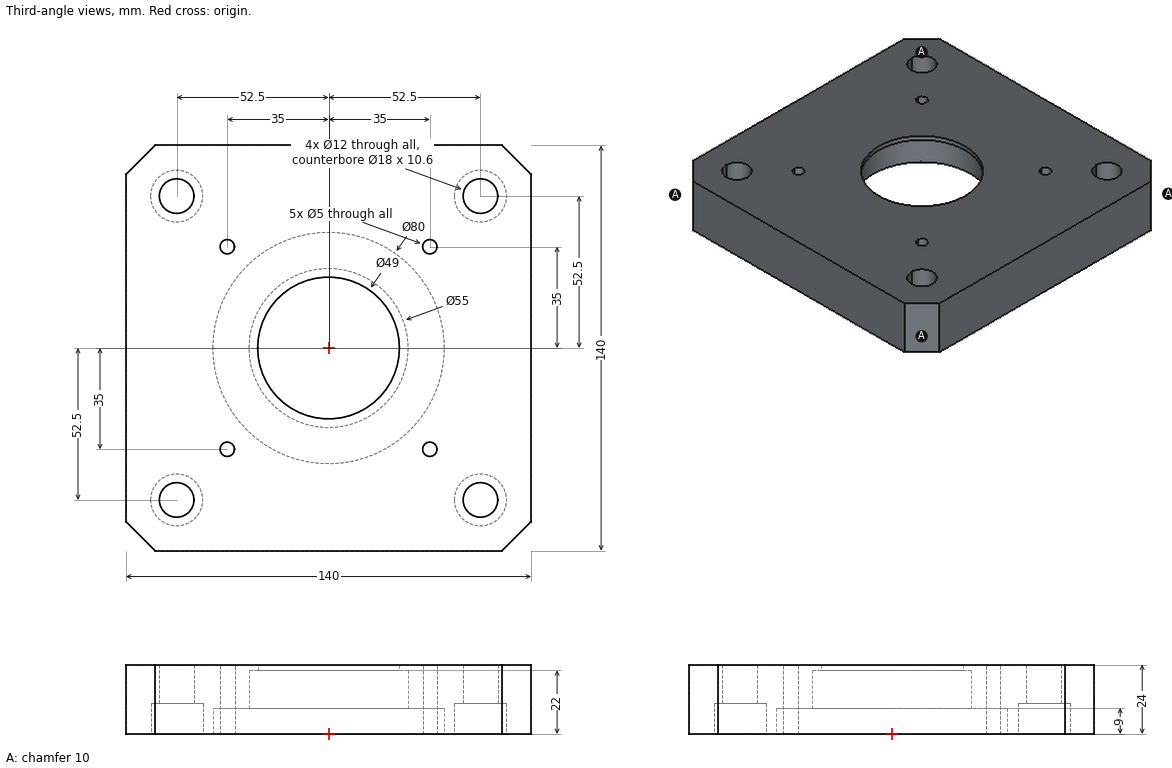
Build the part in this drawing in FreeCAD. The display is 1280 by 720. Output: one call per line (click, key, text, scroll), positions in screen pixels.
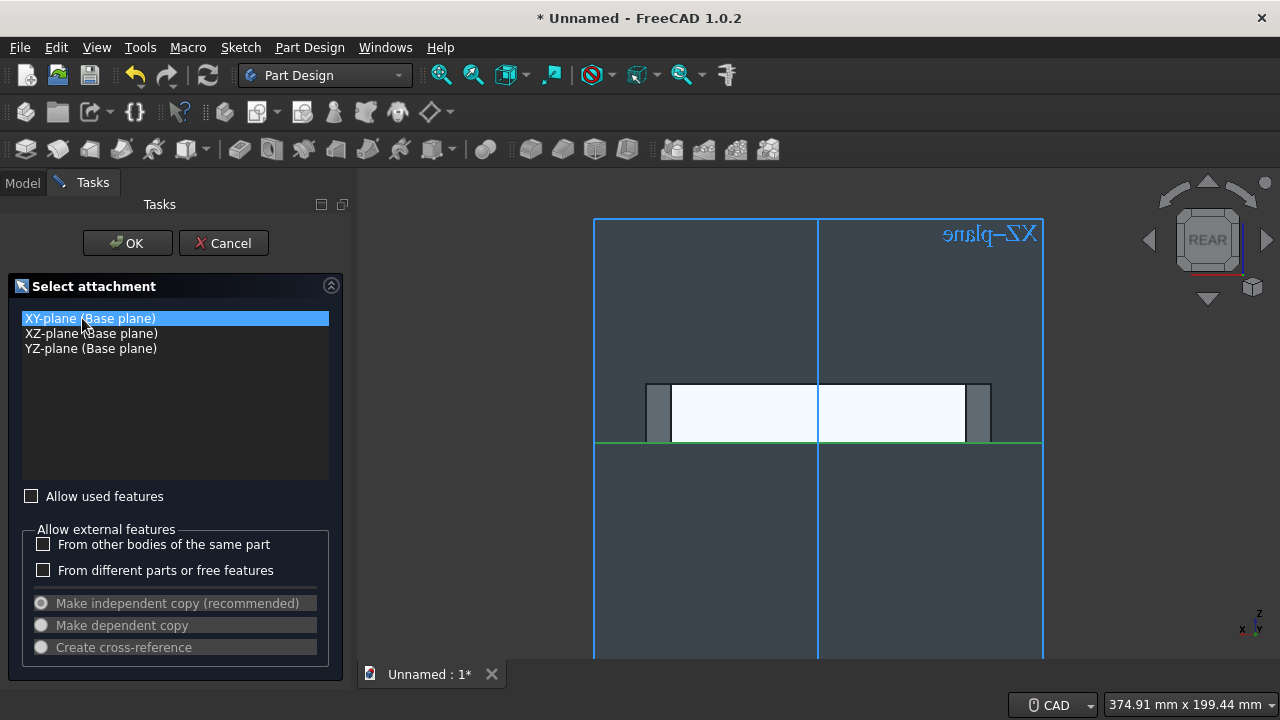
click(128, 243)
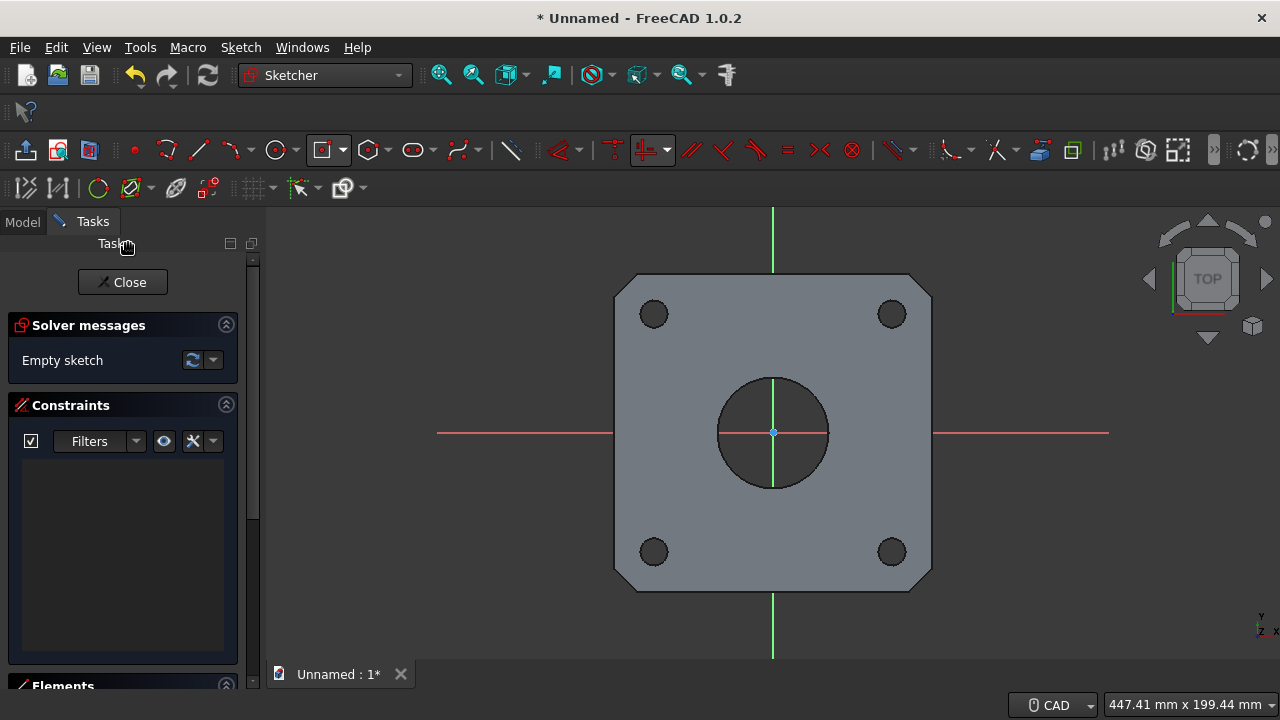
click(90, 150)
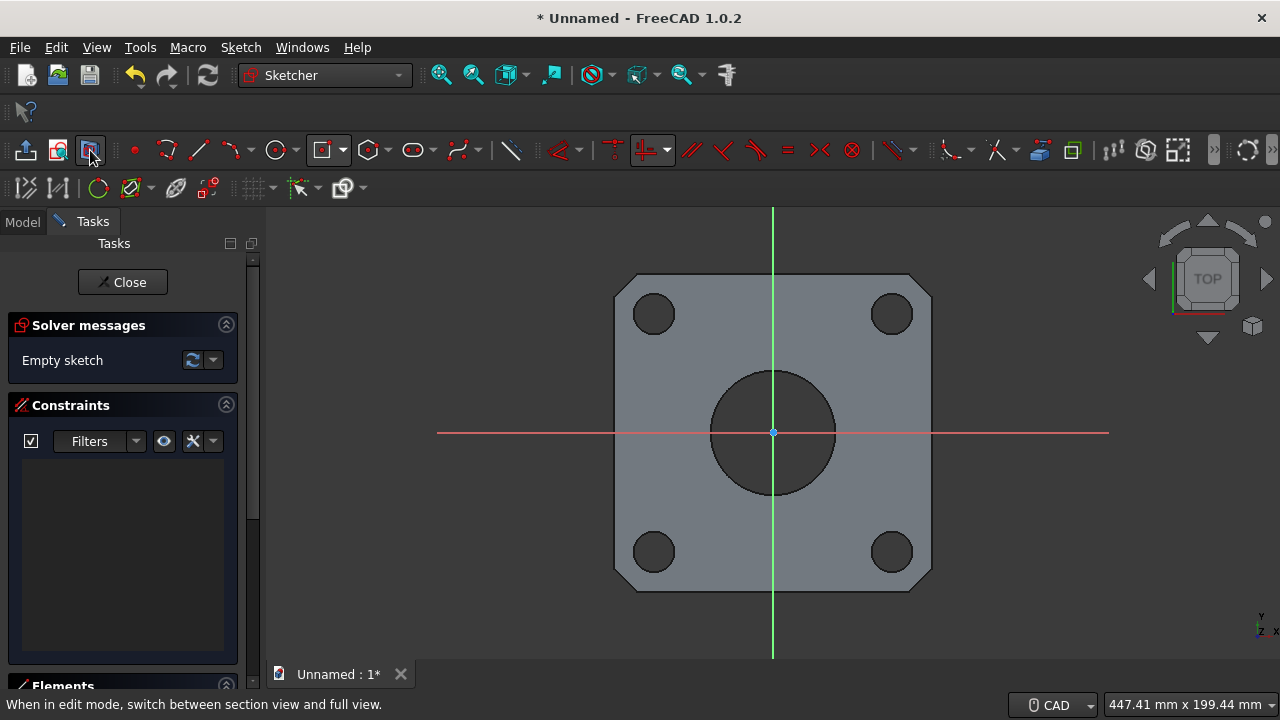
scroll(912, 433, up, 2)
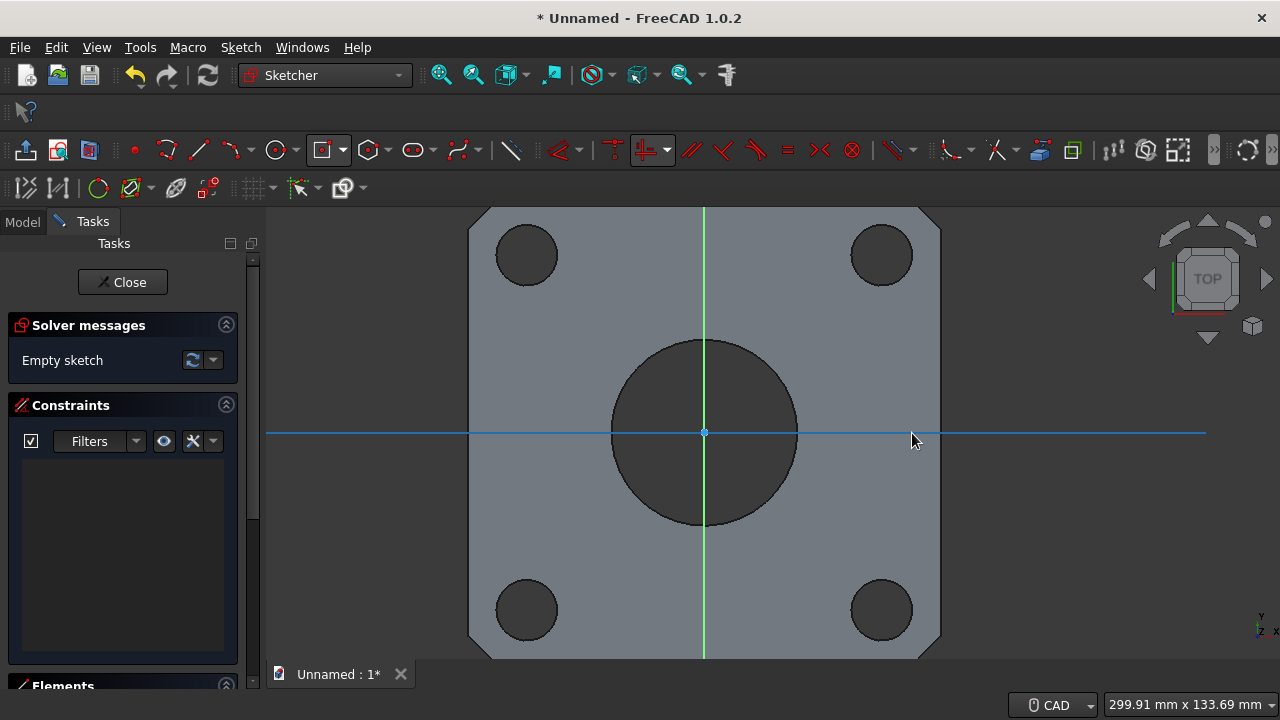
click(276, 150)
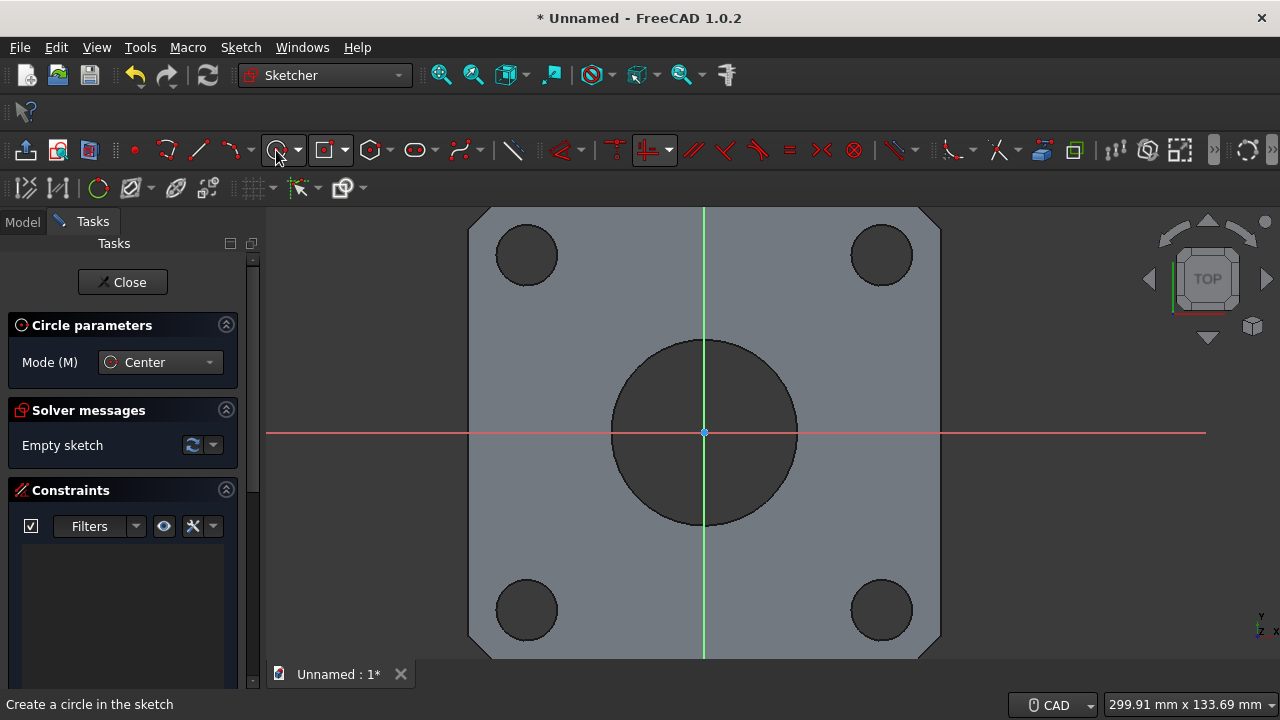
scroll(823, 314, up, 5)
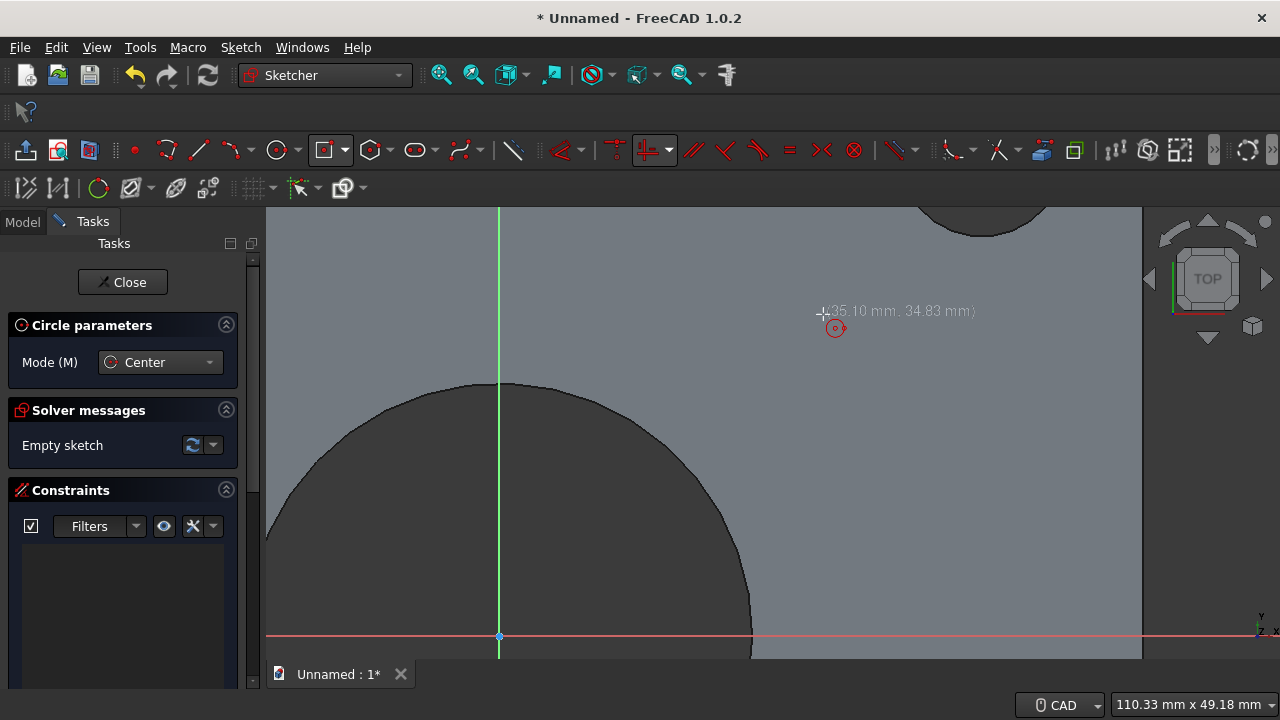
click(821, 315)
move(837, 298)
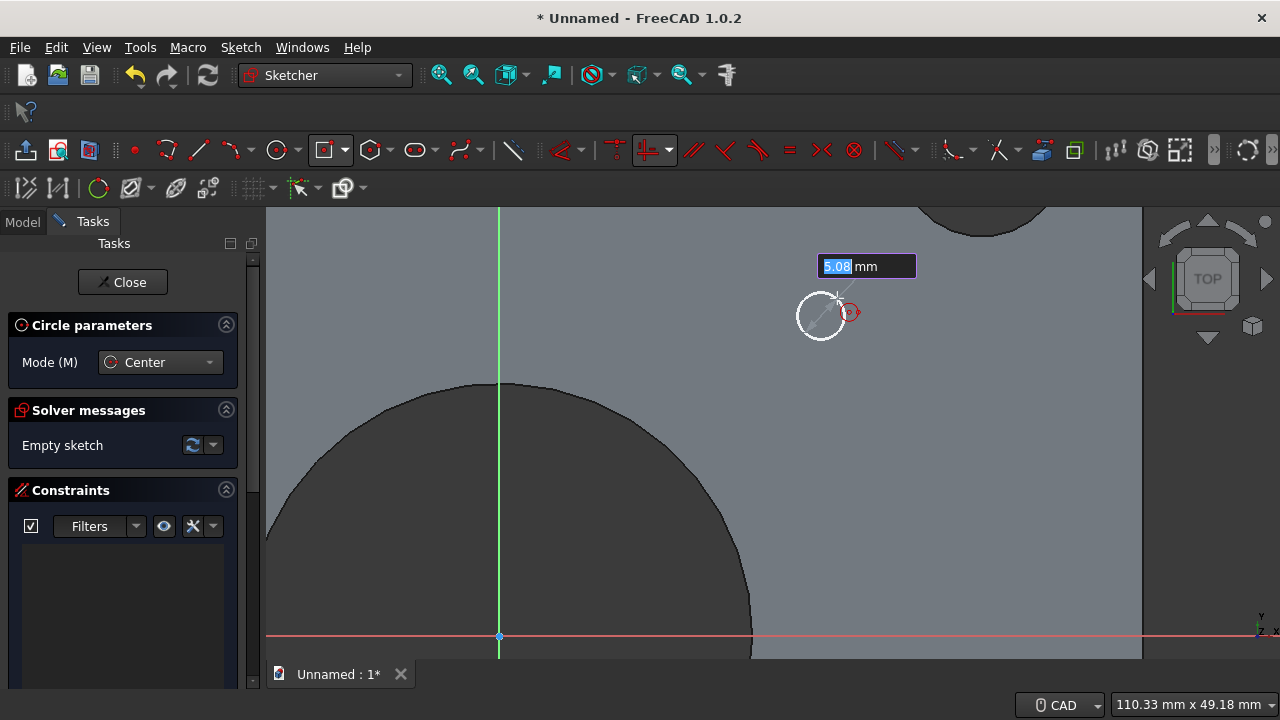
text(5)
key(Return)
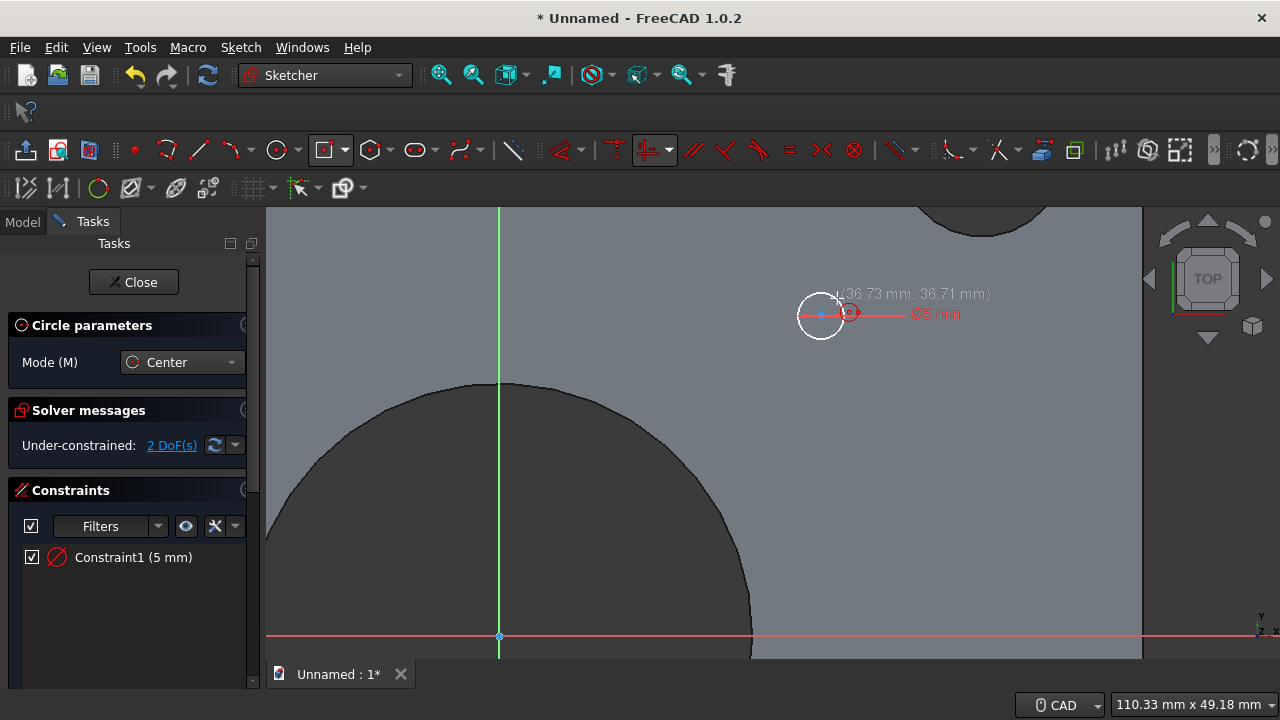
scroll(824, 315, down, 5)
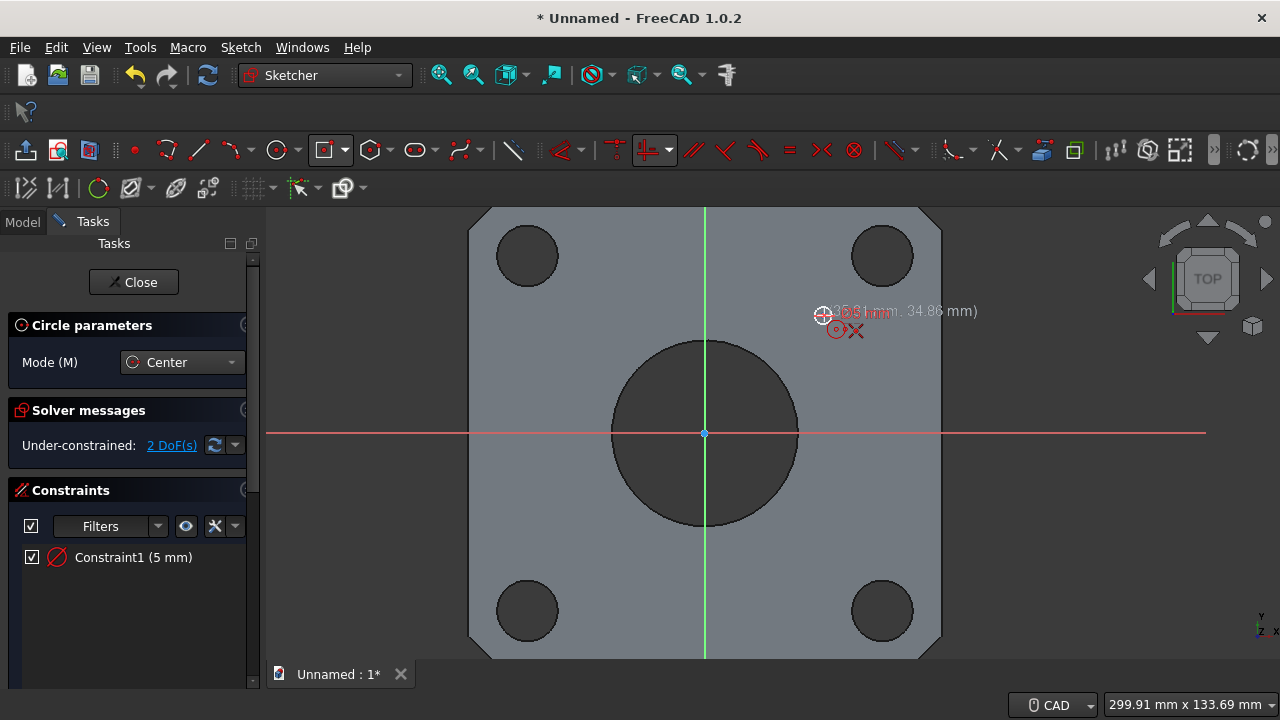
scroll(587, 315, up, 5)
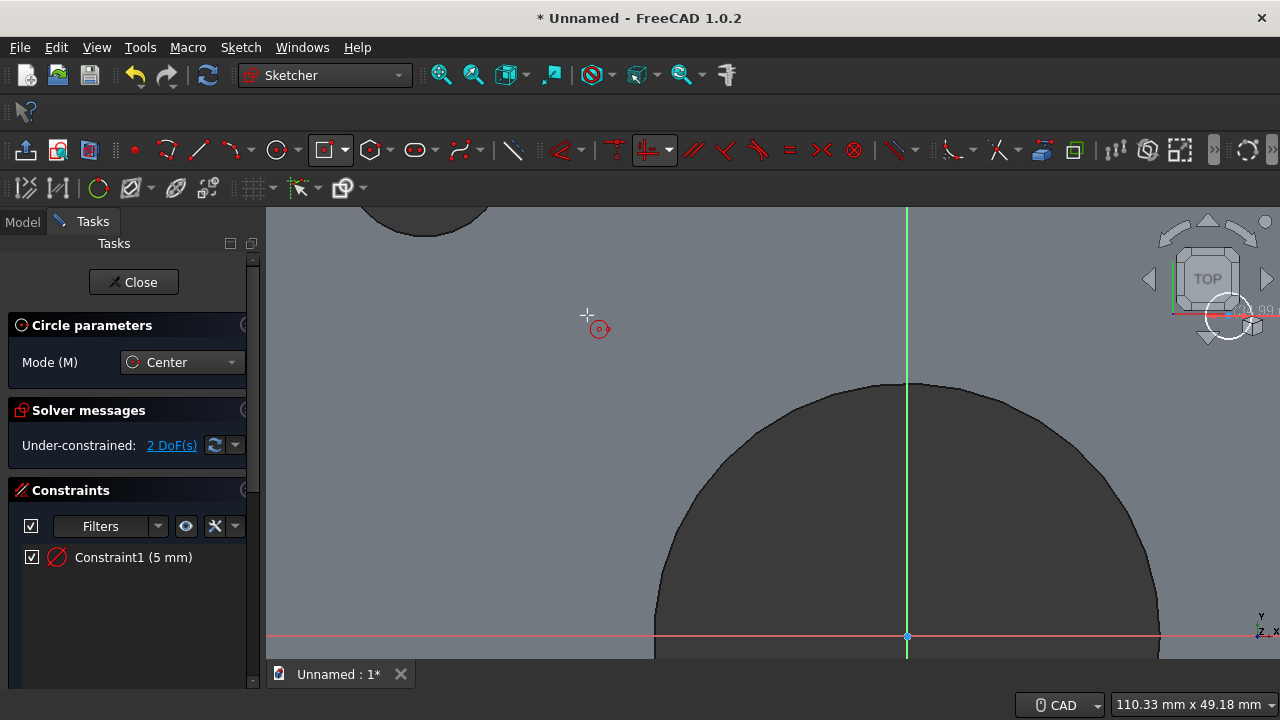
click(585, 315)
move(602, 298)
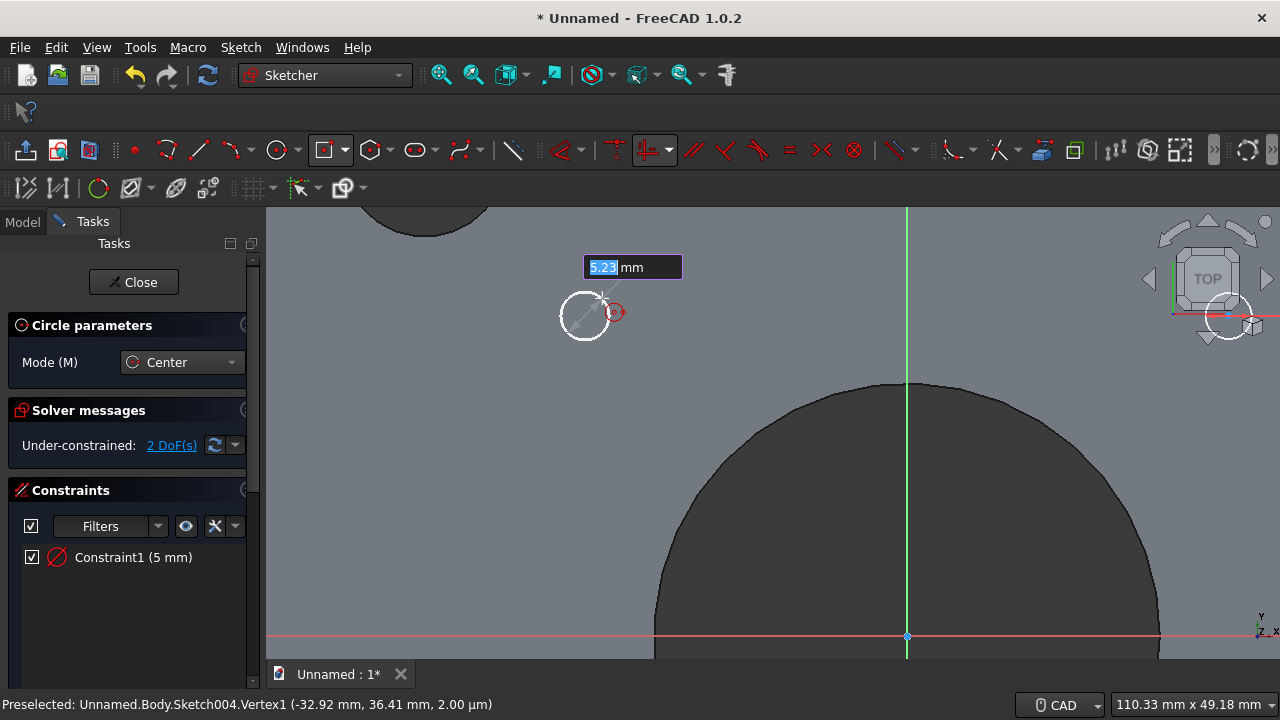
text(5)
key(Return)